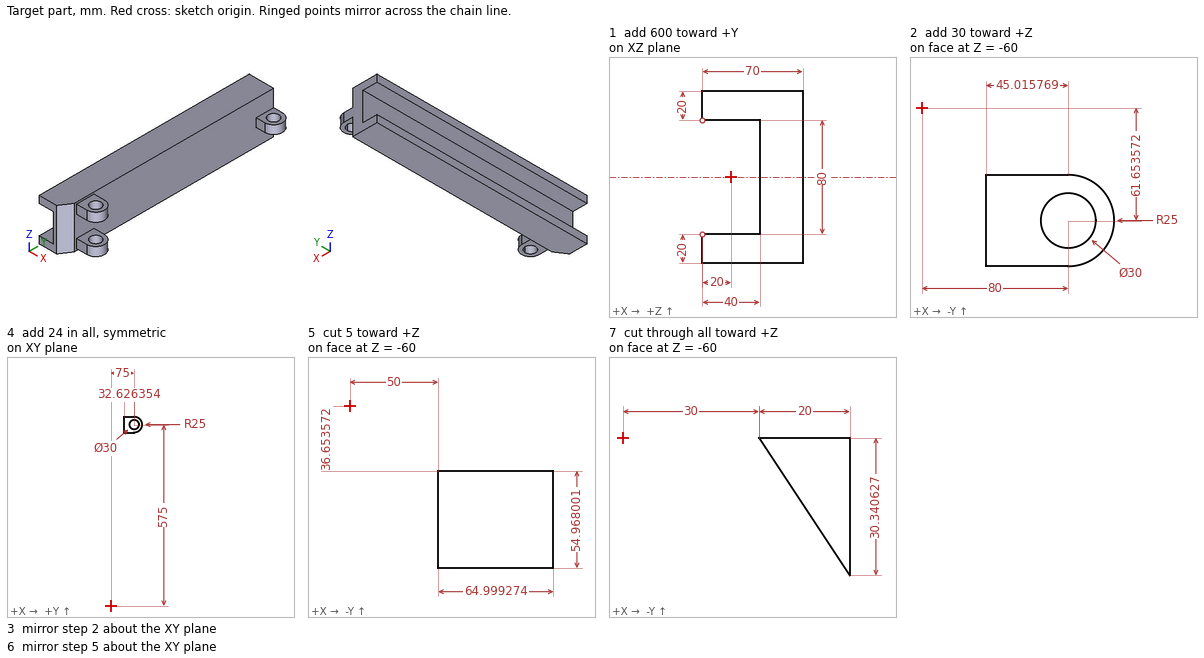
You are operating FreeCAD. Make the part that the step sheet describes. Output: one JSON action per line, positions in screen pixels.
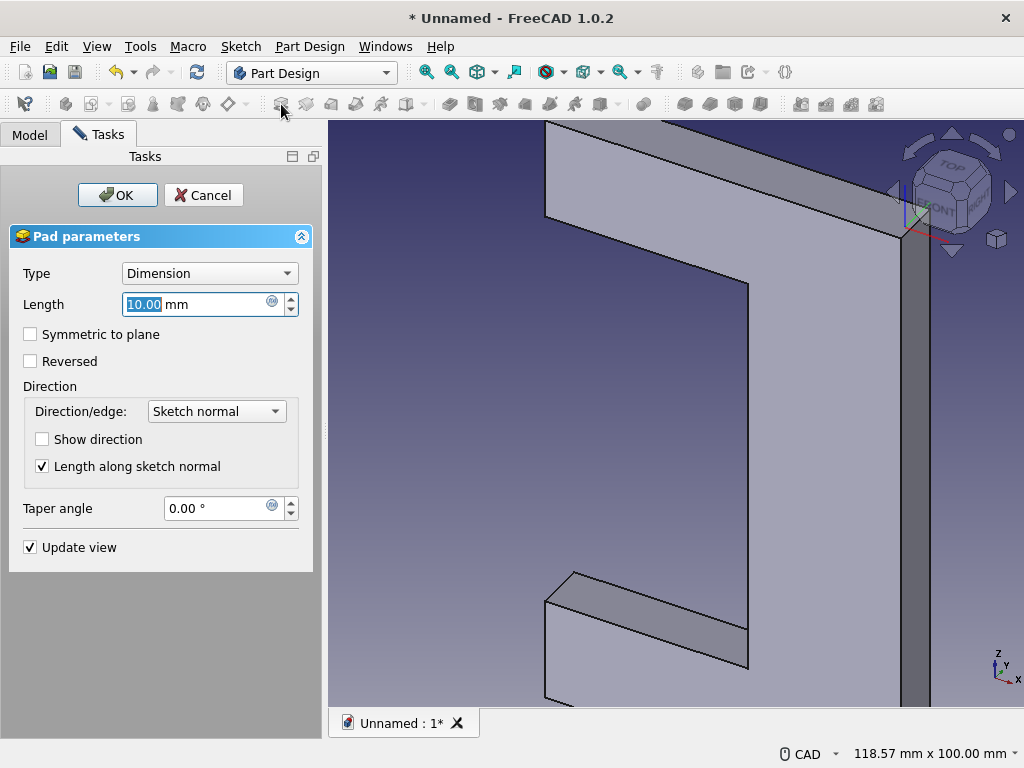
{"action": "type", "text": "600"}
{"action": "key", "text": "Tab"}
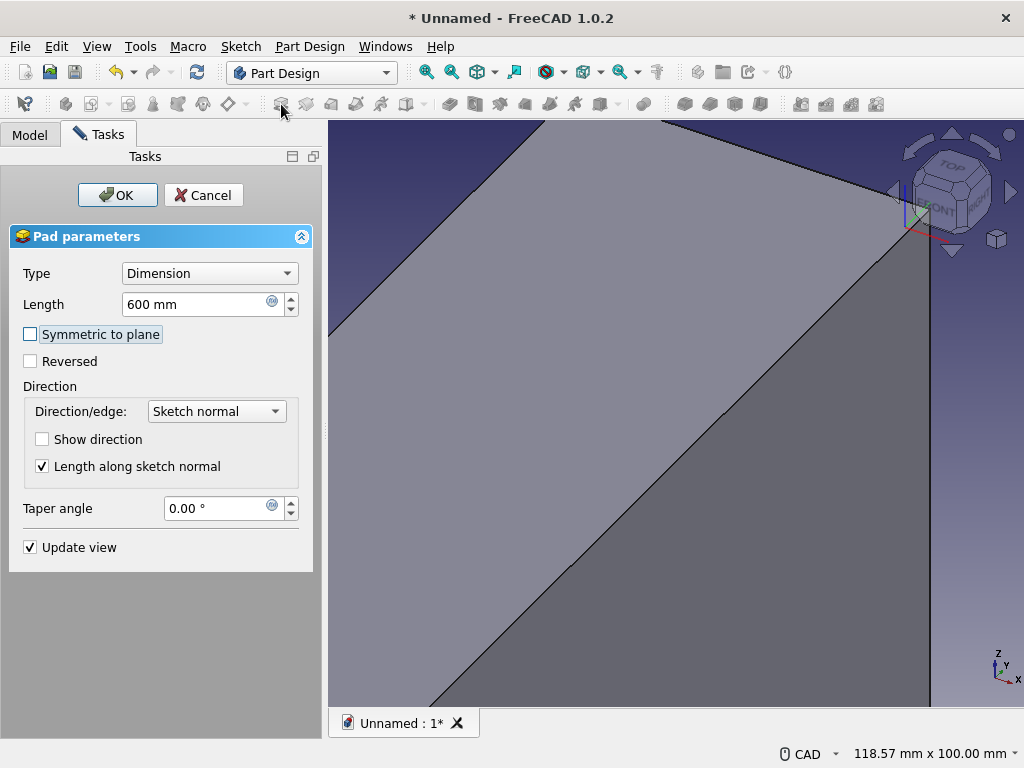
{"action": "left_click", "coordinate": [31, 361]}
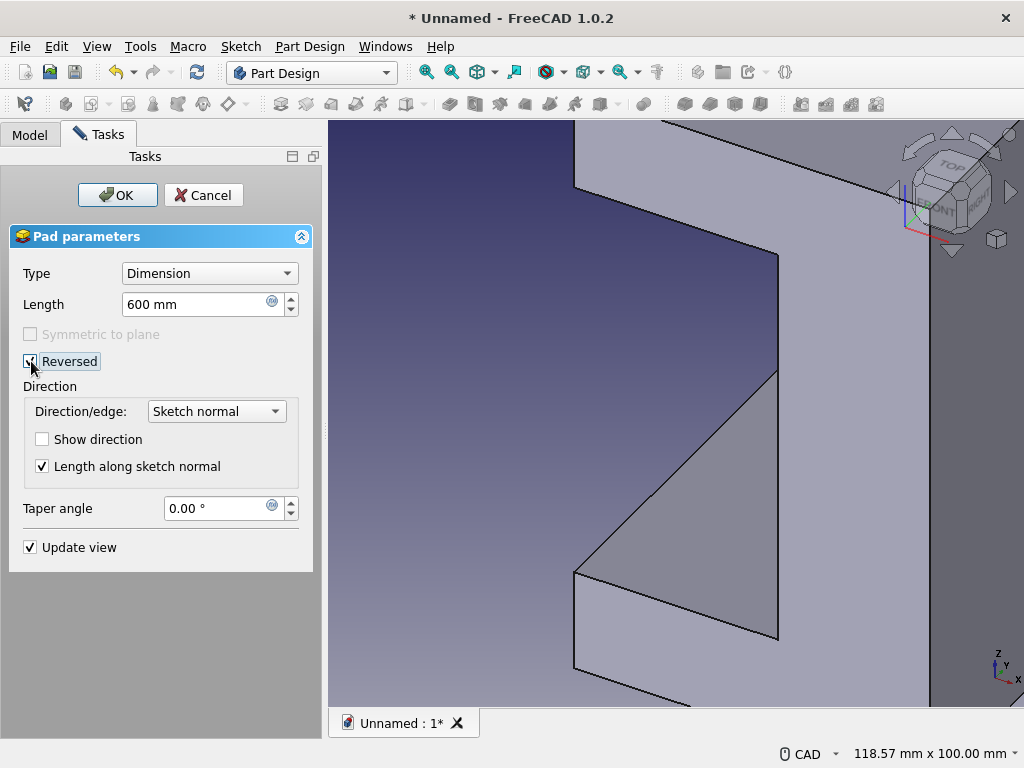
{"action": "left_click", "coordinate": [118, 195]}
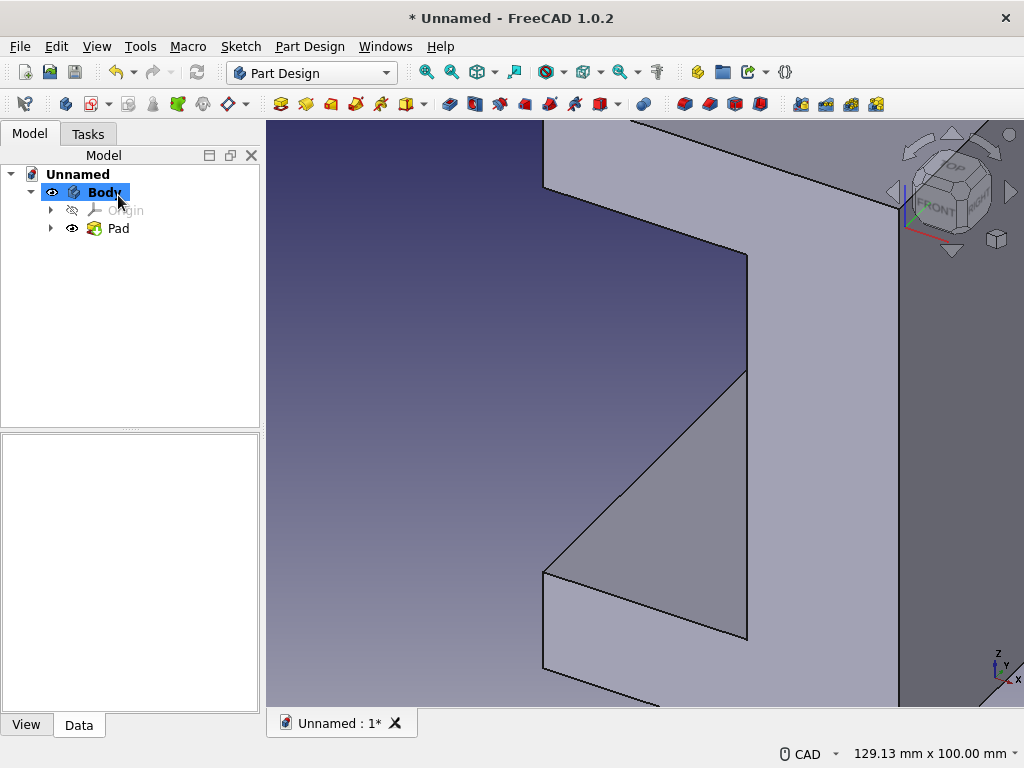
{"action": "left_click", "coordinate": [427, 72]}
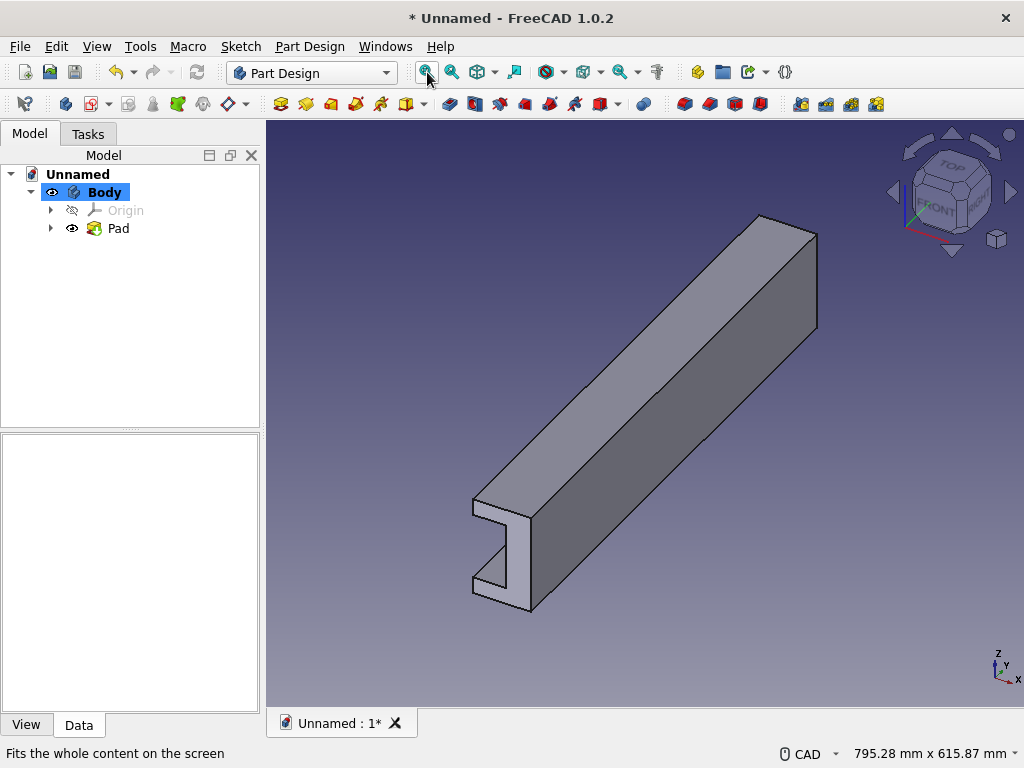
{"action": "key", "text": "5"}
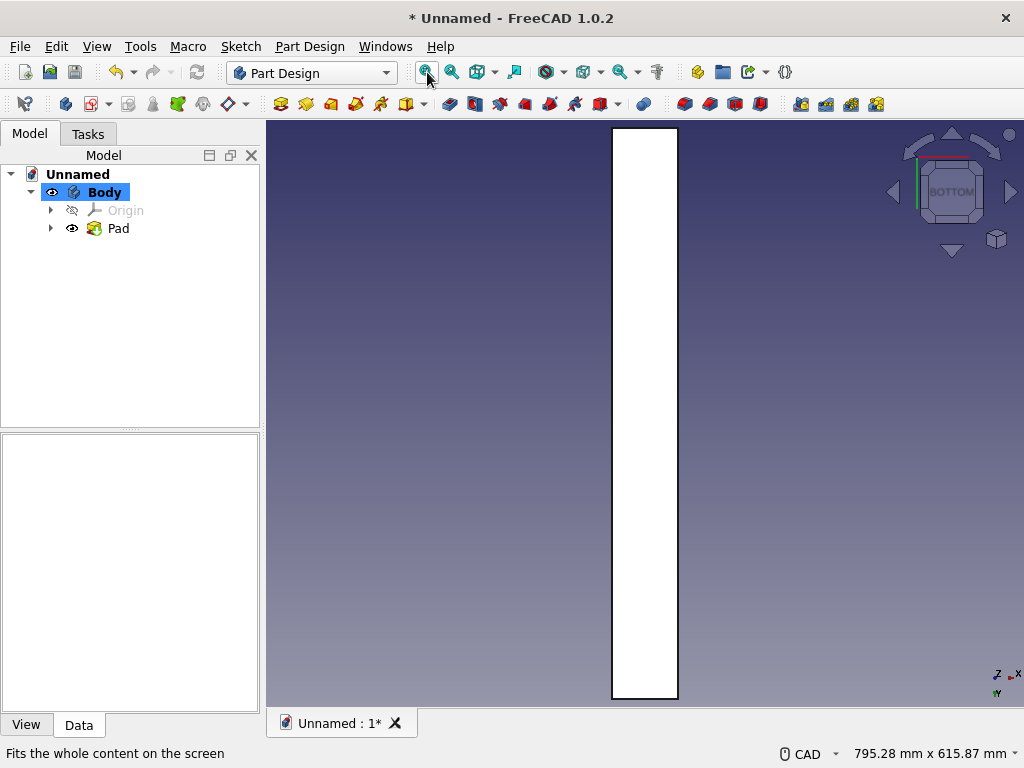
{"action": "left_click", "coordinate": [645, 658]}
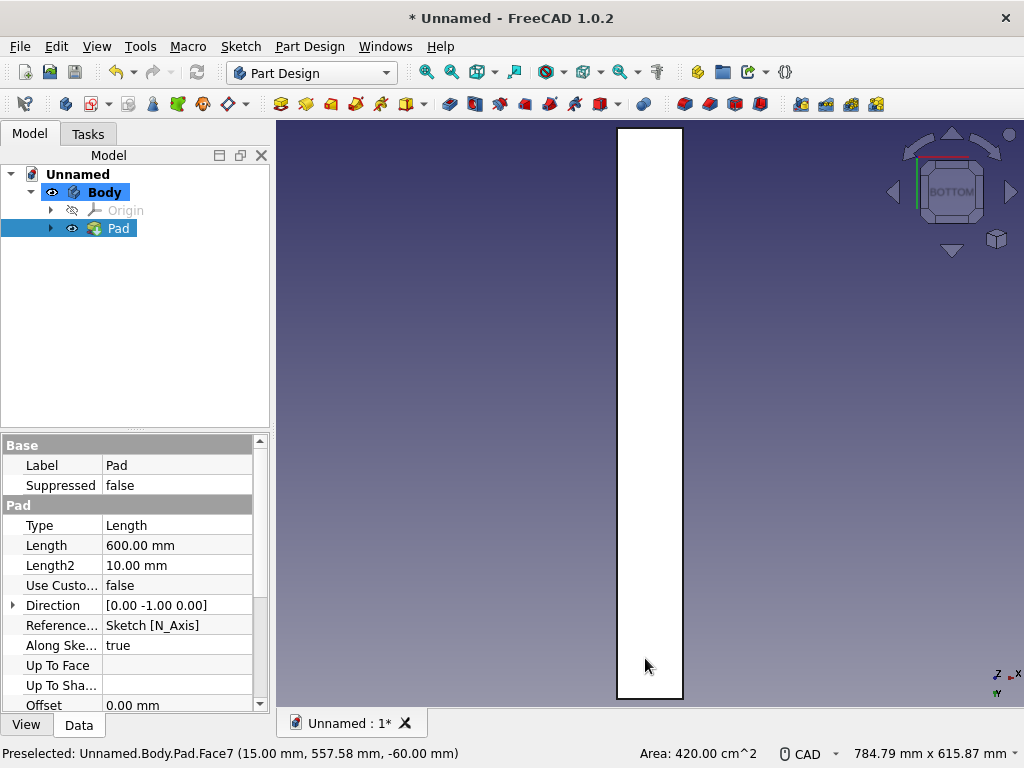
{"action": "left_click", "coordinate": [90, 104]}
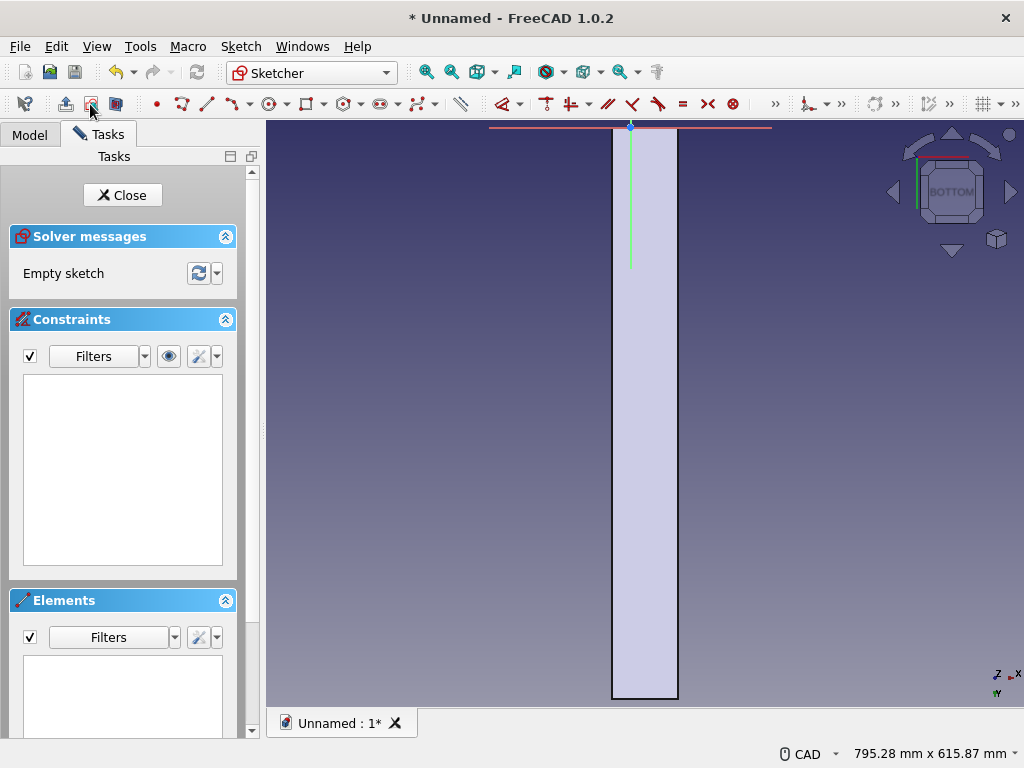
{"action": "scroll", "coordinate": [576, 414], "scroll_direction": "down", "scroll_amount": 5}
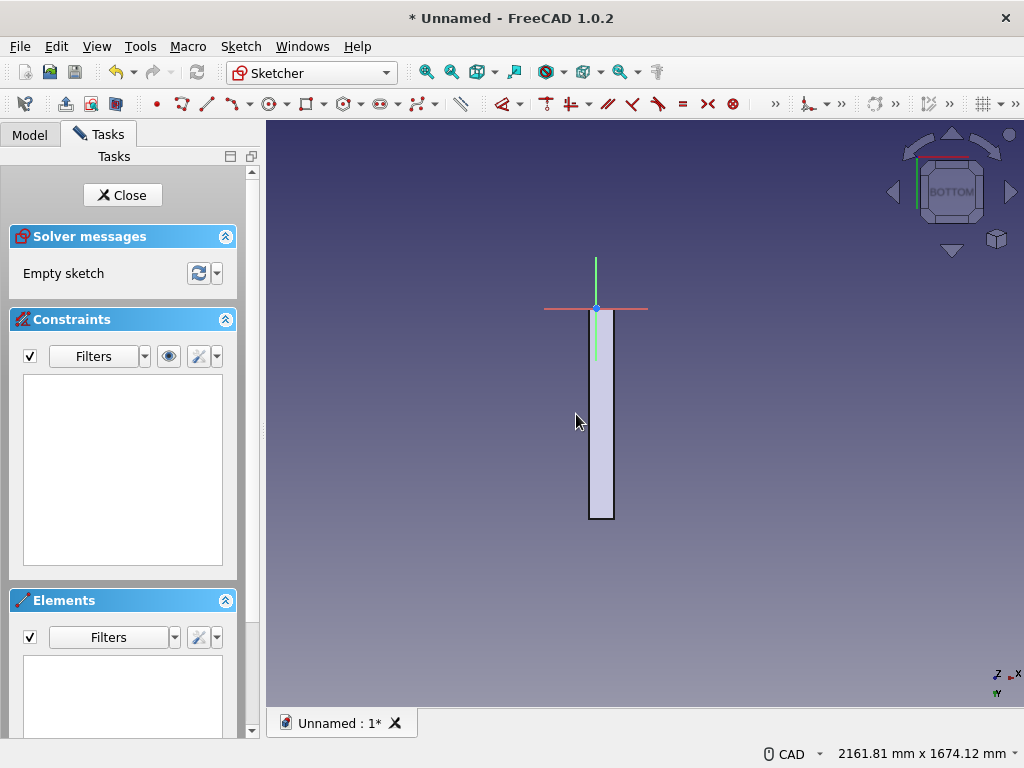
{"action": "scroll", "coordinate": [619, 315], "scroll_direction": "up", "scroll_amount": 12}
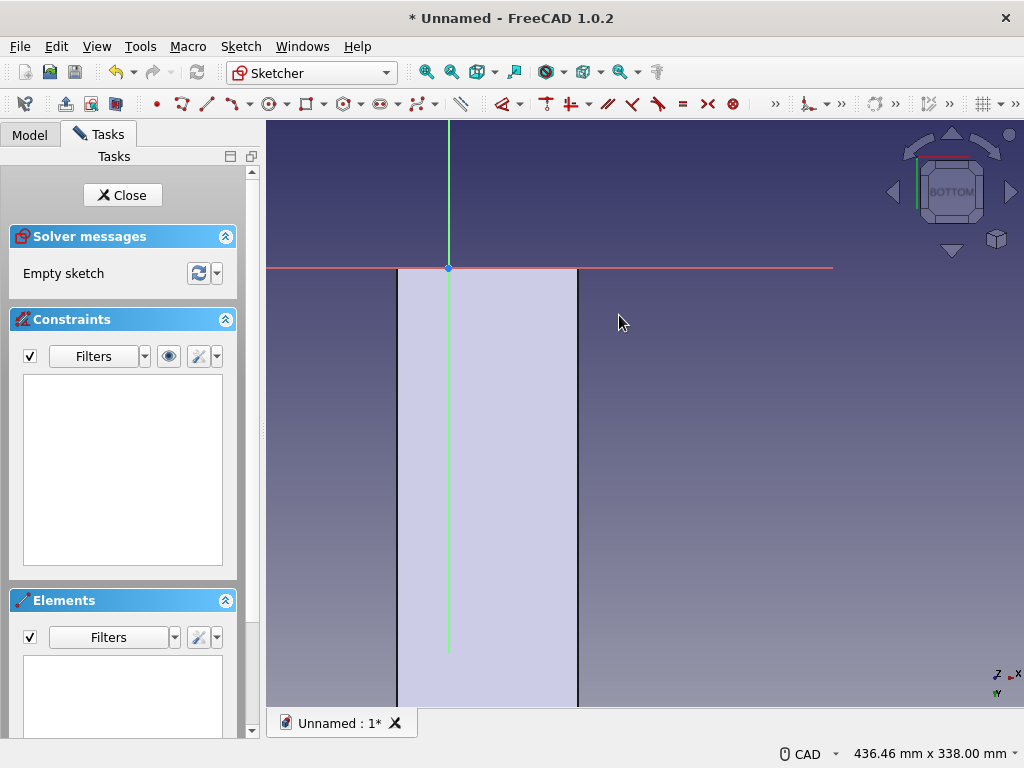
{"action": "left_click", "coordinate": [182, 104]}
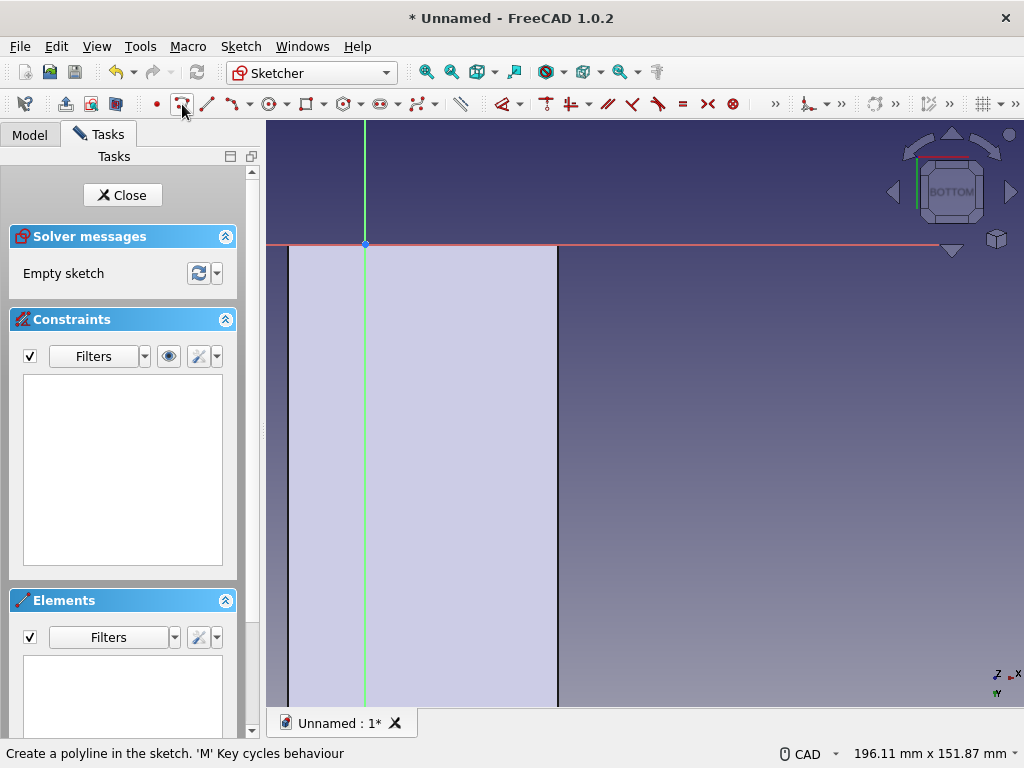
{"action": "left_click", "coordinate": [674, 387]}
{"action": "left_click", "coordinate": [500, 387]}
{"action": "left_click", "coordinate": [500, 580]}
{"action": "left_click", "coordinate": [674, 580]}
{"action": "right_click", "coordinate": [674, 580]}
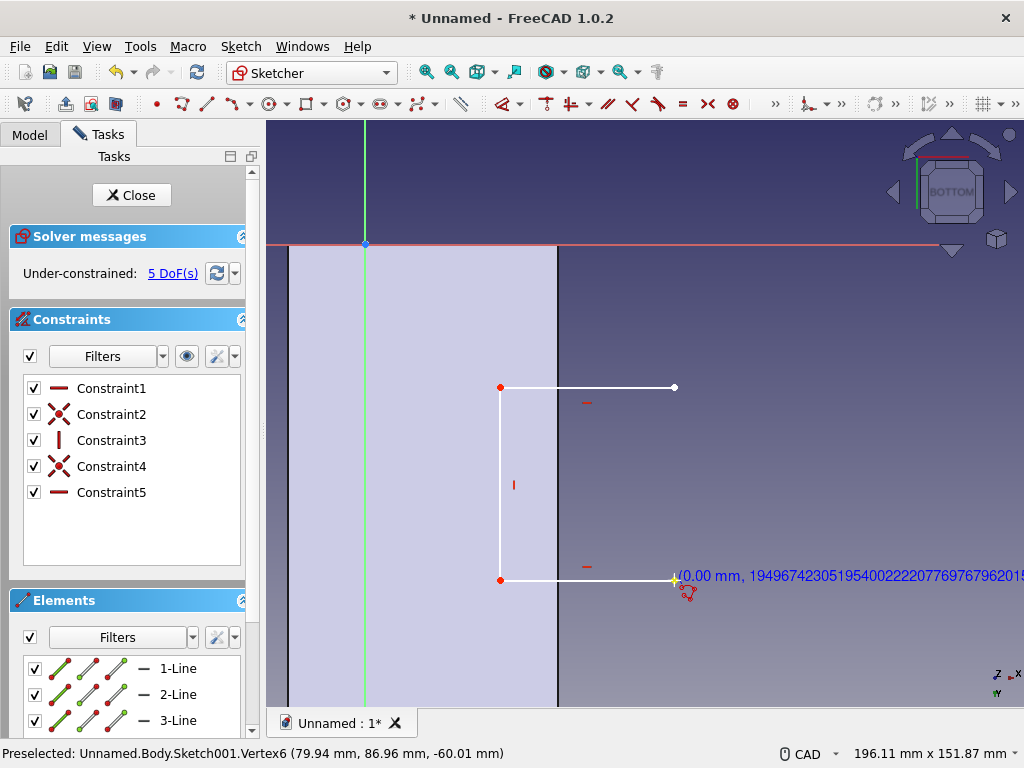
{"action": "left_click", "coordinate": [232, 104]}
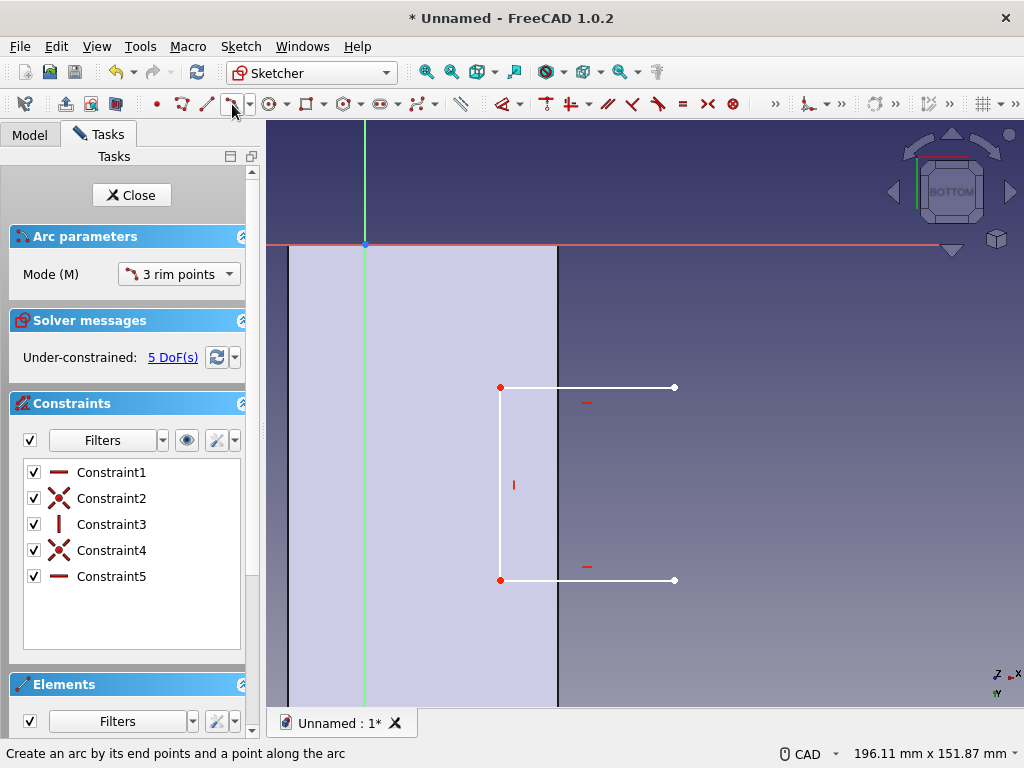
{"action": "left_click", "coordinate": [674, 581]}
{"action": "left_click", "coordinate": [674, 388]}
{"action": "left_click", "coordinate": [771, 483]}